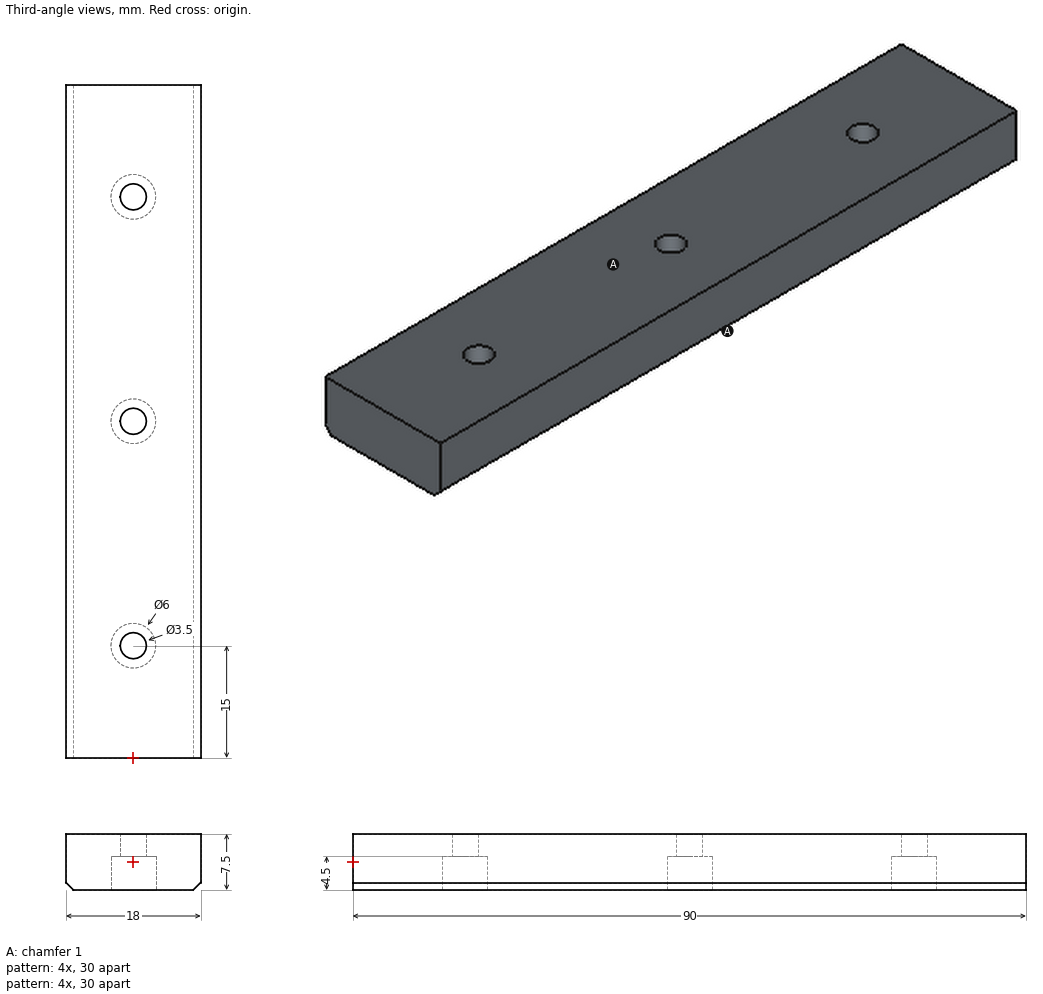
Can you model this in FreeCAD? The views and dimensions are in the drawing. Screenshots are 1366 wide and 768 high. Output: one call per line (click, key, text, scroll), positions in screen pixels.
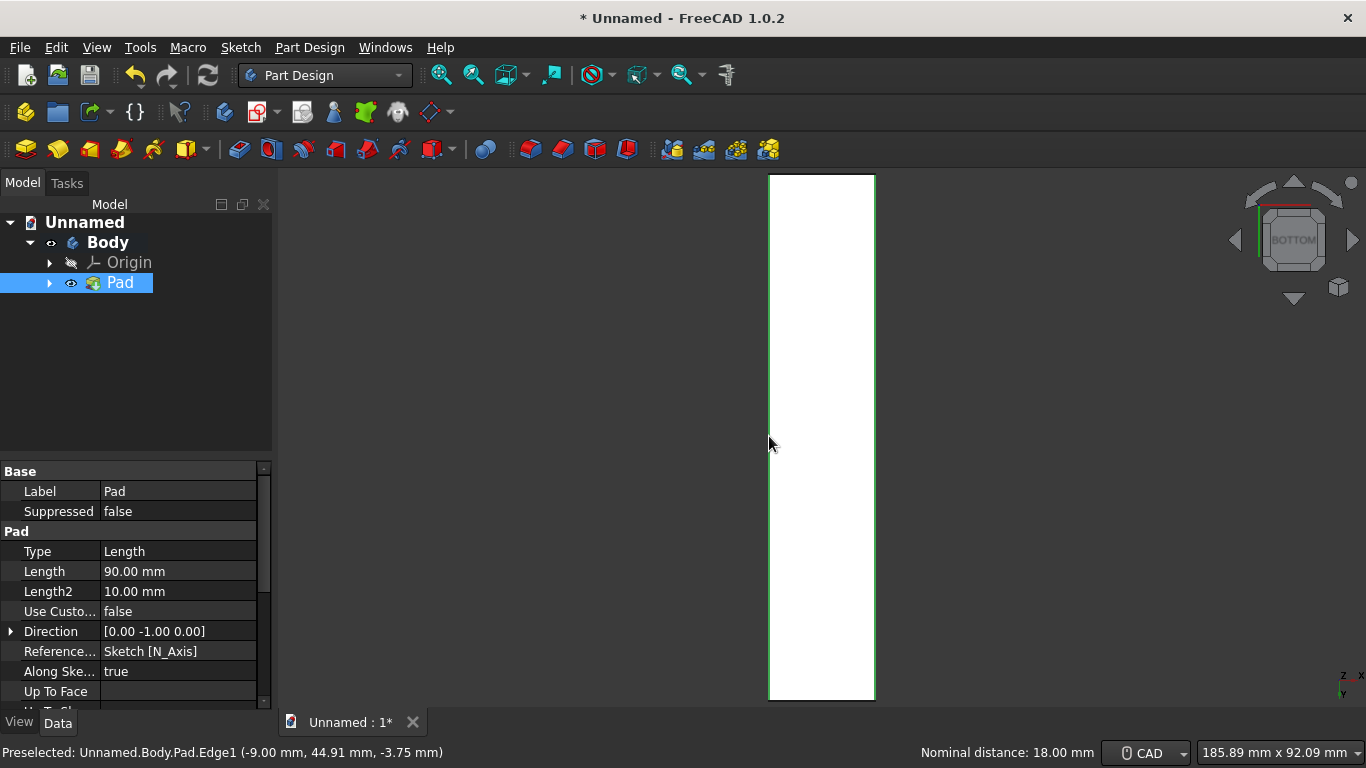
click(564, 150)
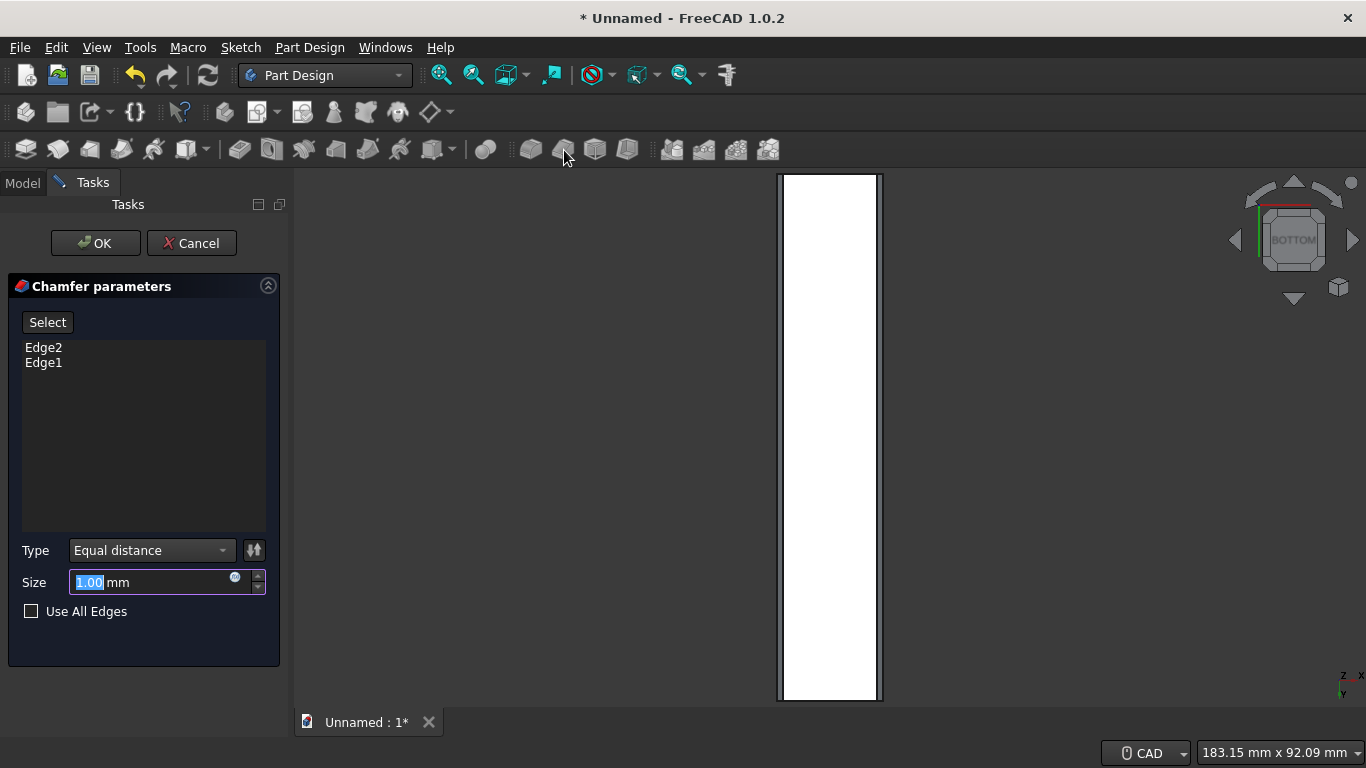
text(1)
key(Tab)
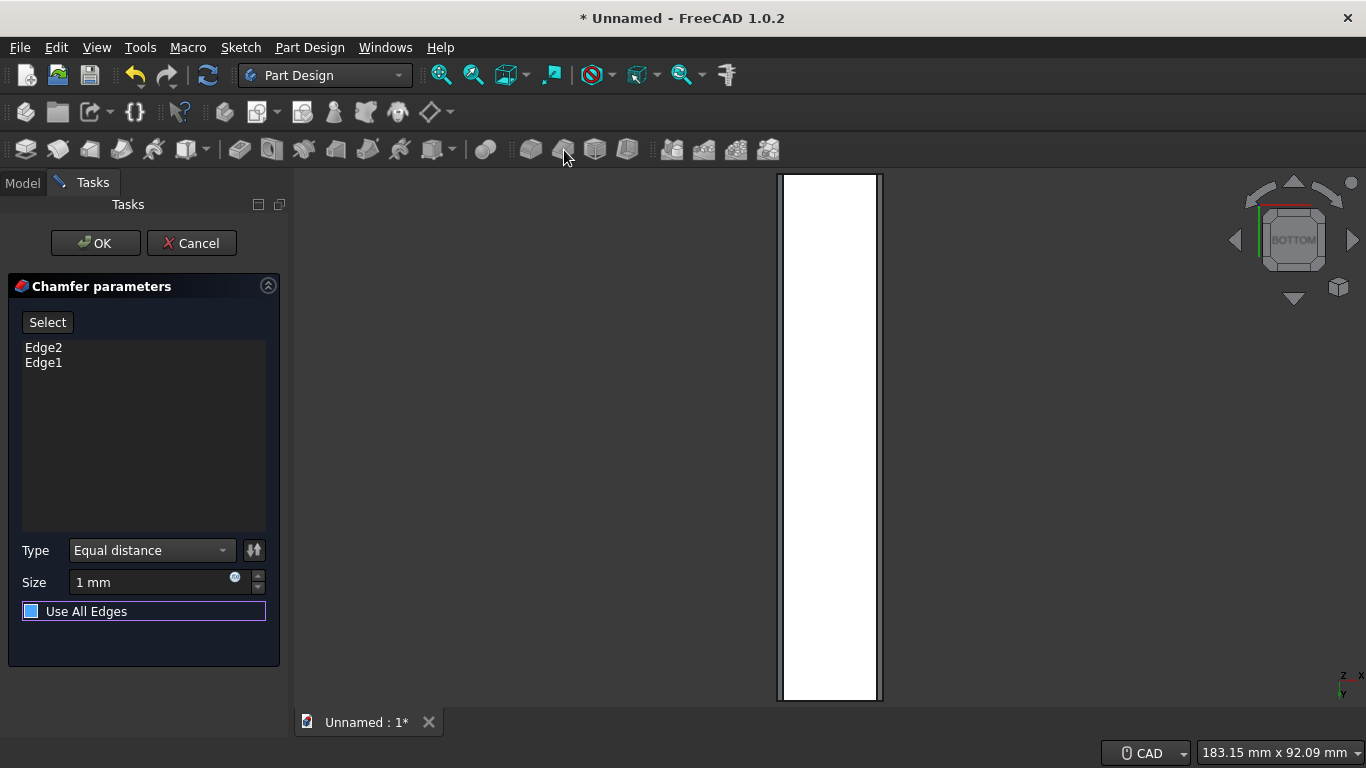
click(96, 243)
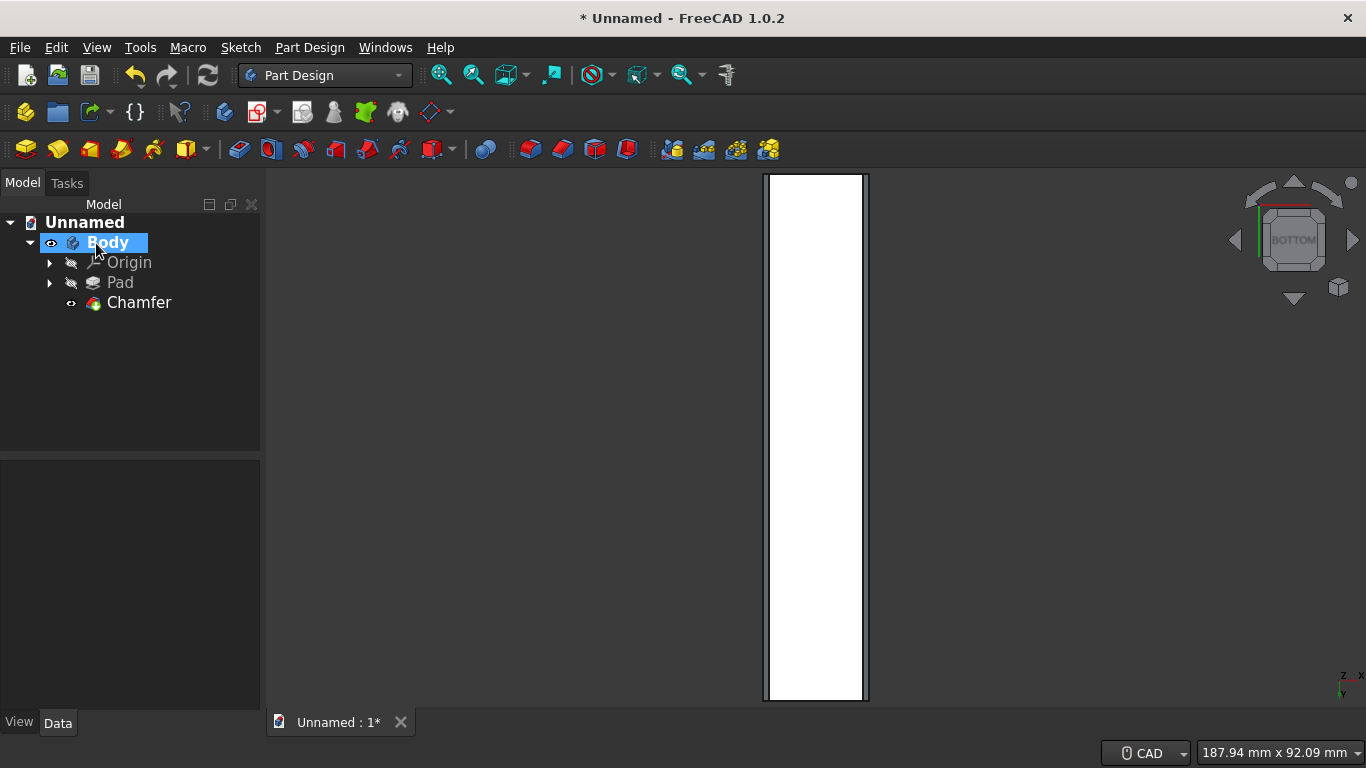
click(816, 587)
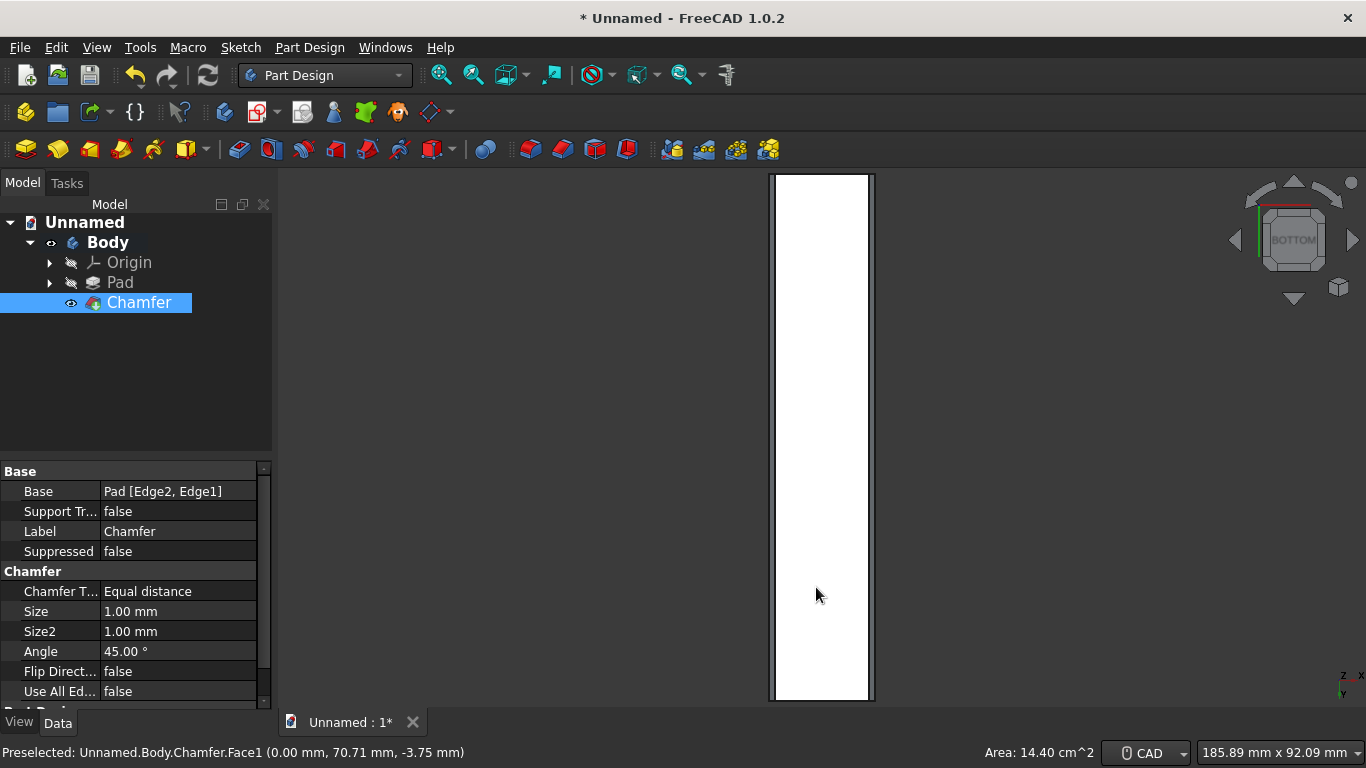
click(258, 112)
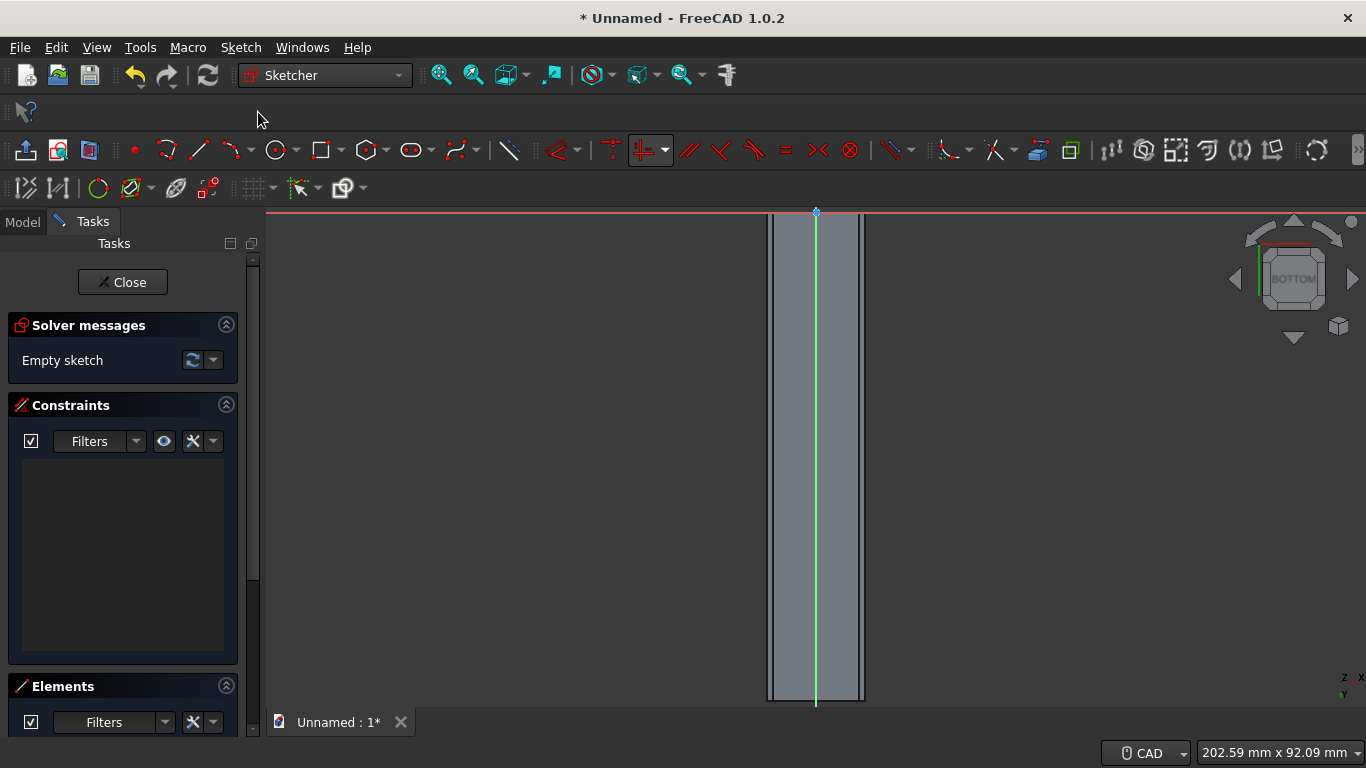
scroll(820, 284, up, 14)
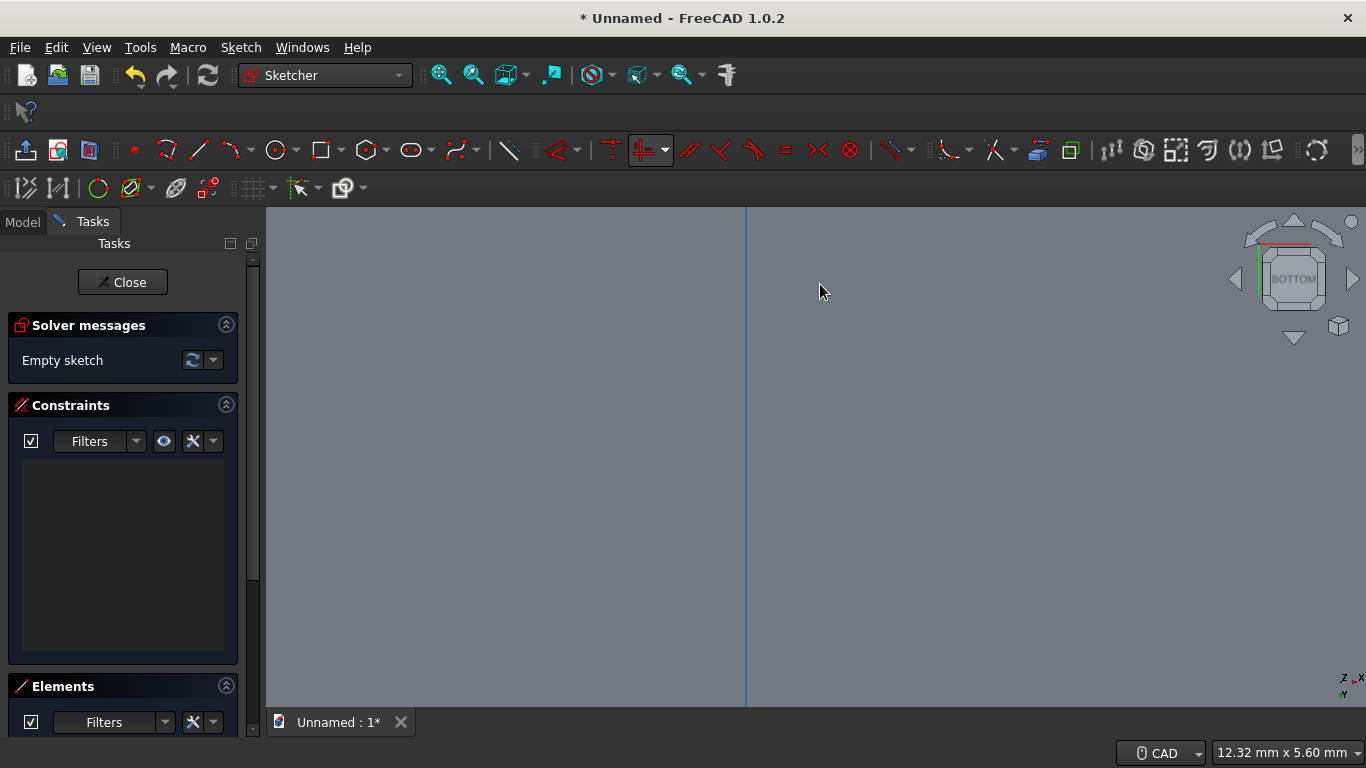
click(276, 150)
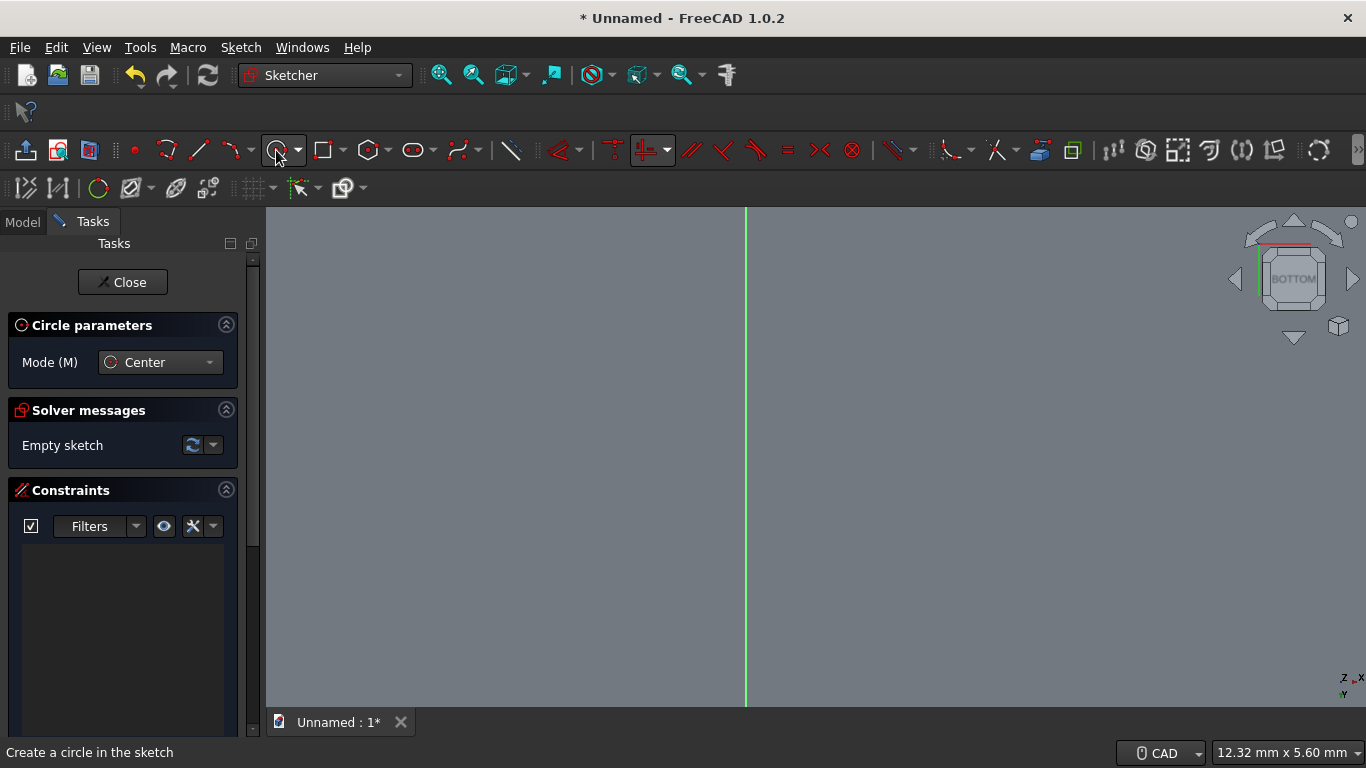
click(746, 448)
click(857, 337)
key(Escape)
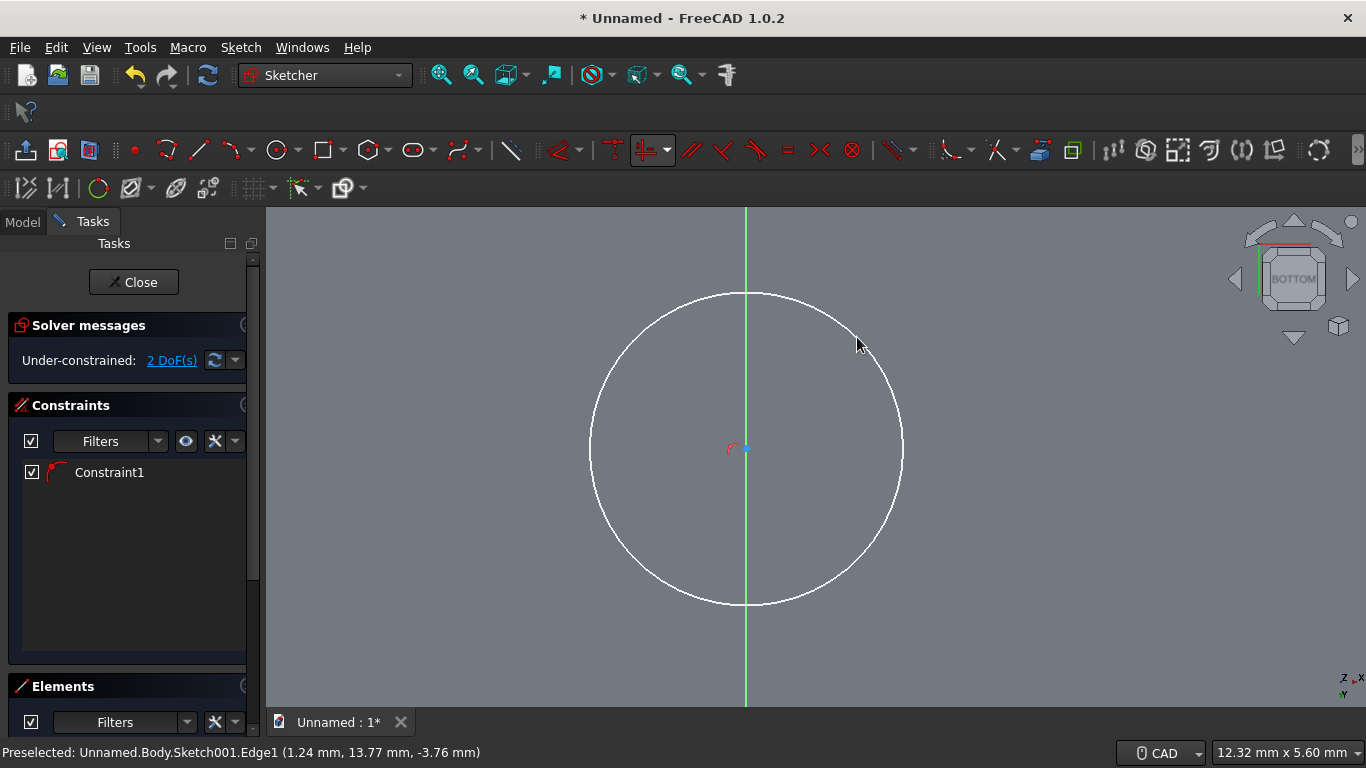
click(857, 338)